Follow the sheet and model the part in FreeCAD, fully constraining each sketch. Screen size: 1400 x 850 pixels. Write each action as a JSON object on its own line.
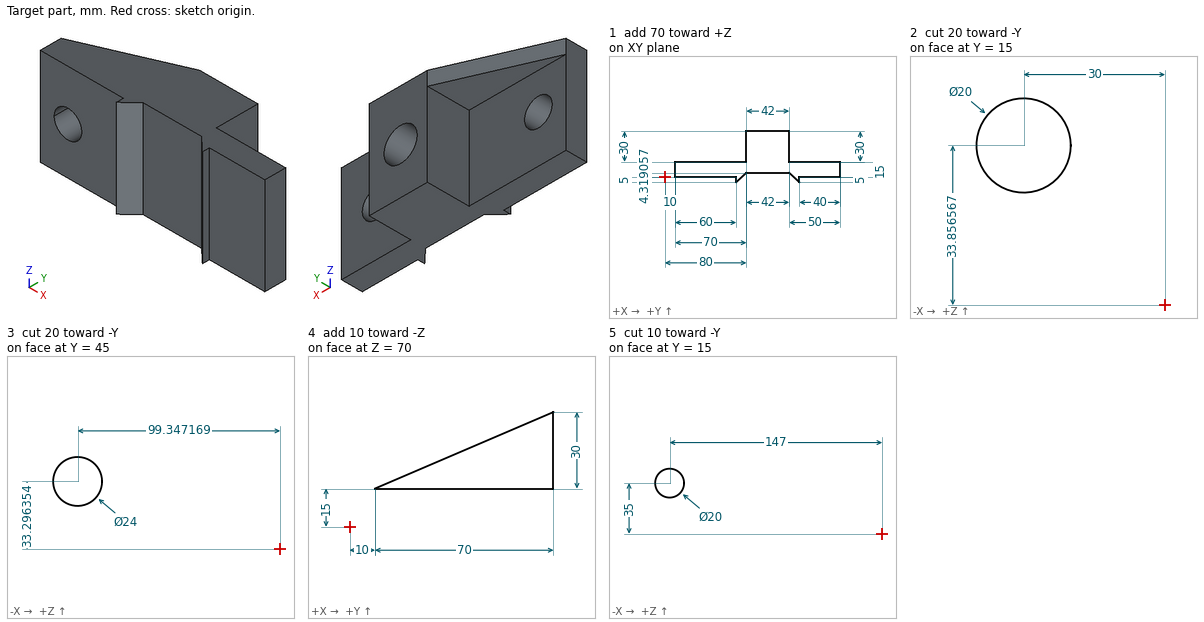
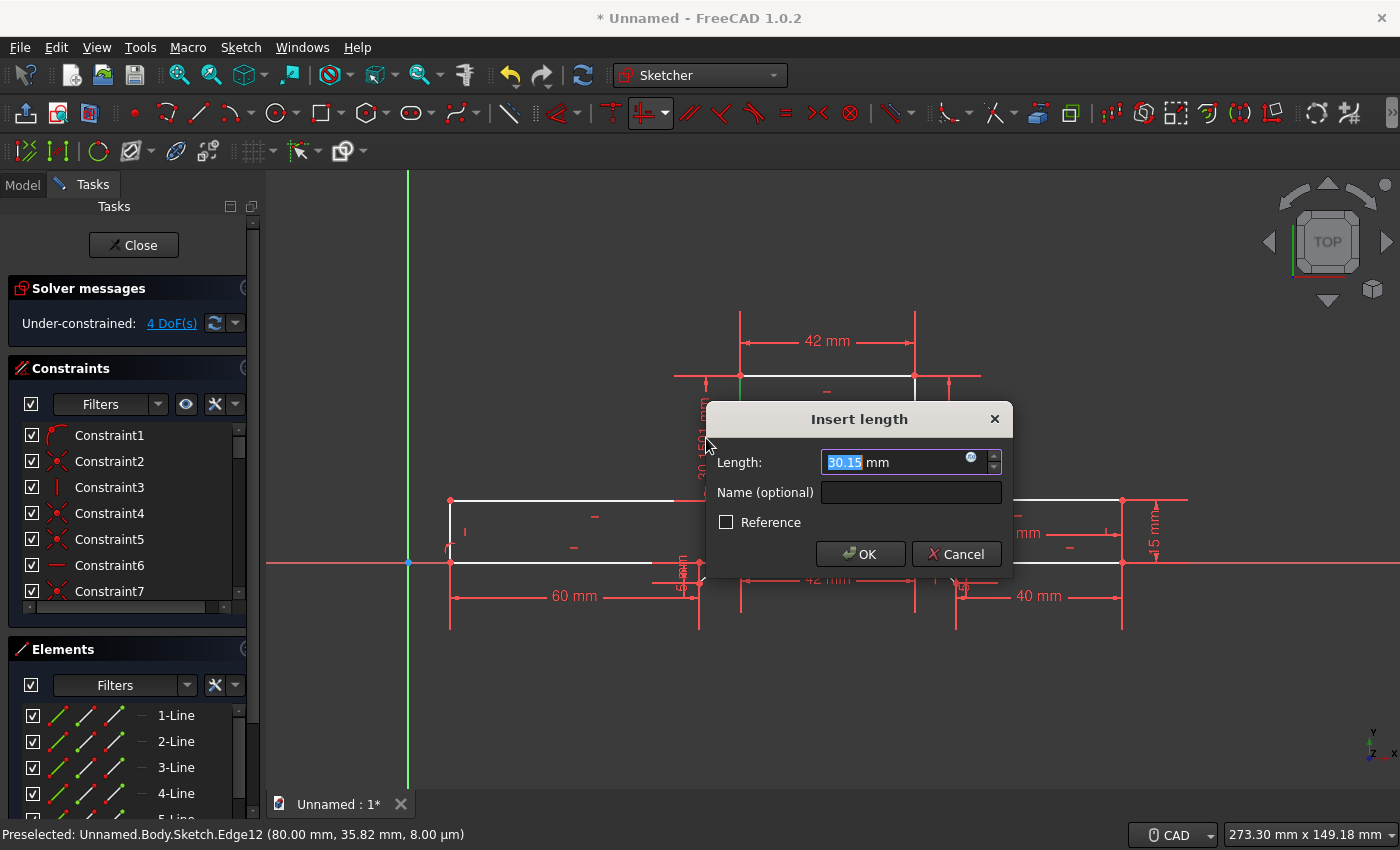
{"action": "type", "text": "30"}
{"action": "key", "text": "Return"}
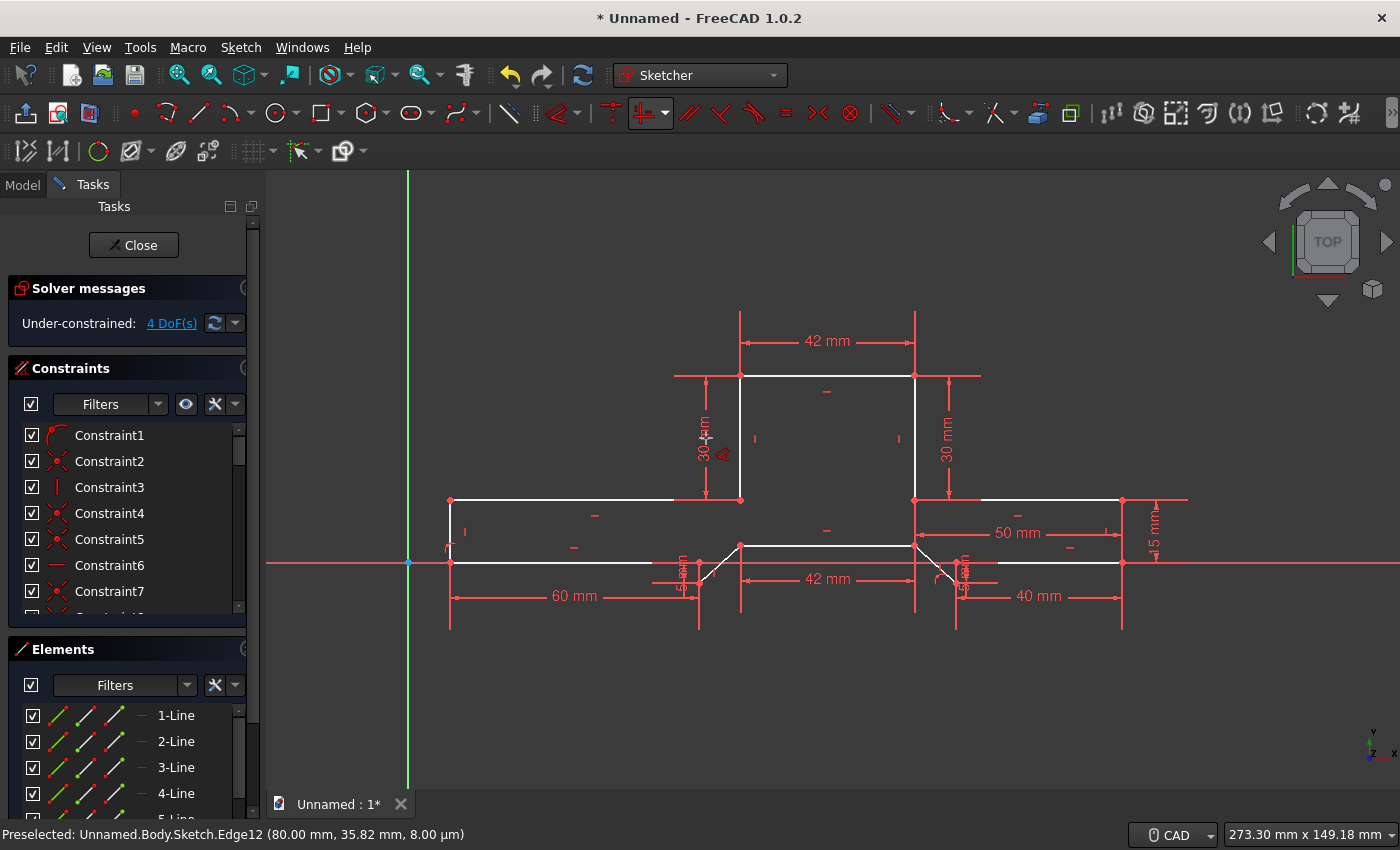
{"action": "left_click", "coordinate": [653, 500]}
{"action": "left_click", "coordinate": [595, 534]}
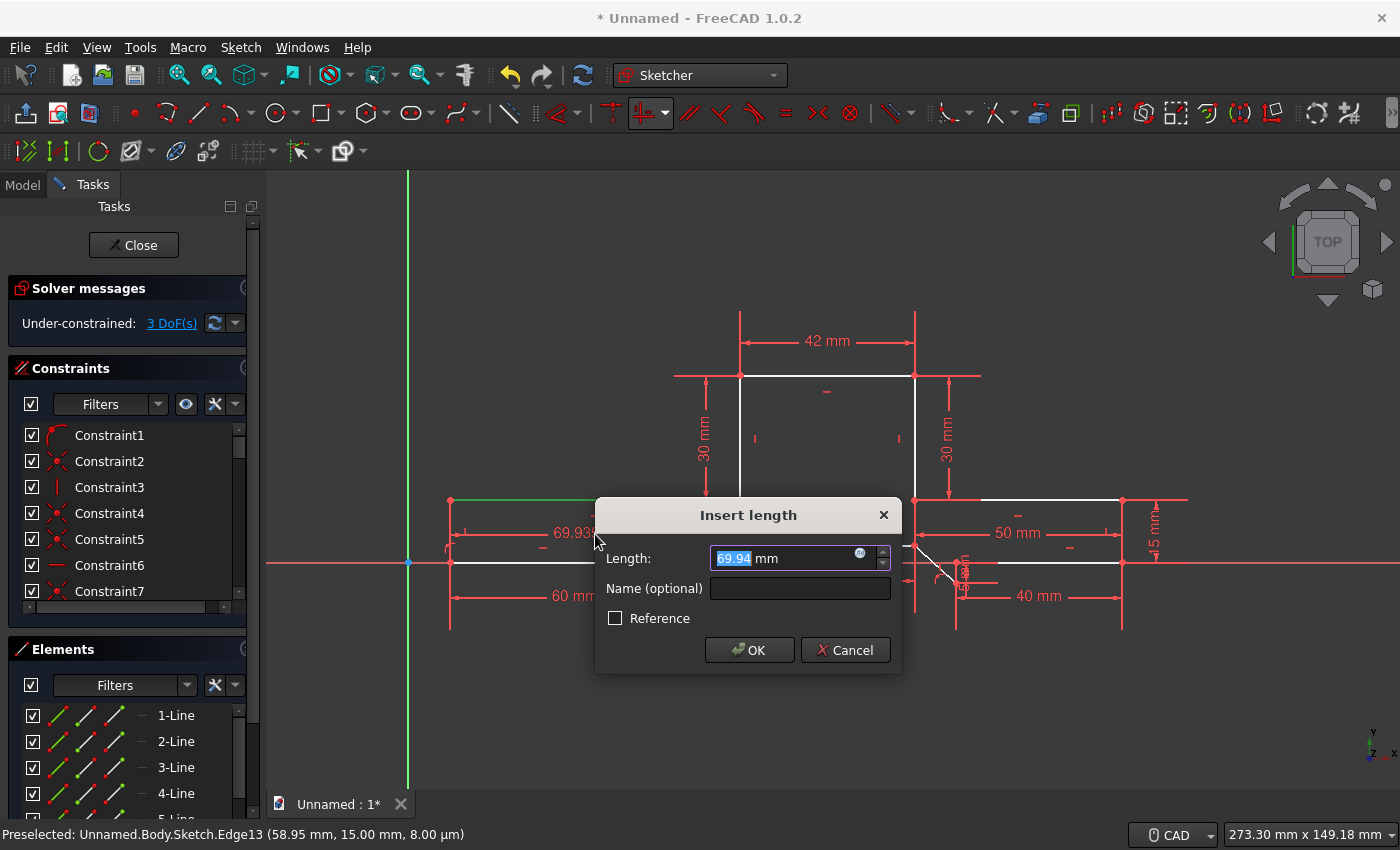
{"action": "type", "text": "70"}
{"action": "key", "text": "Return"}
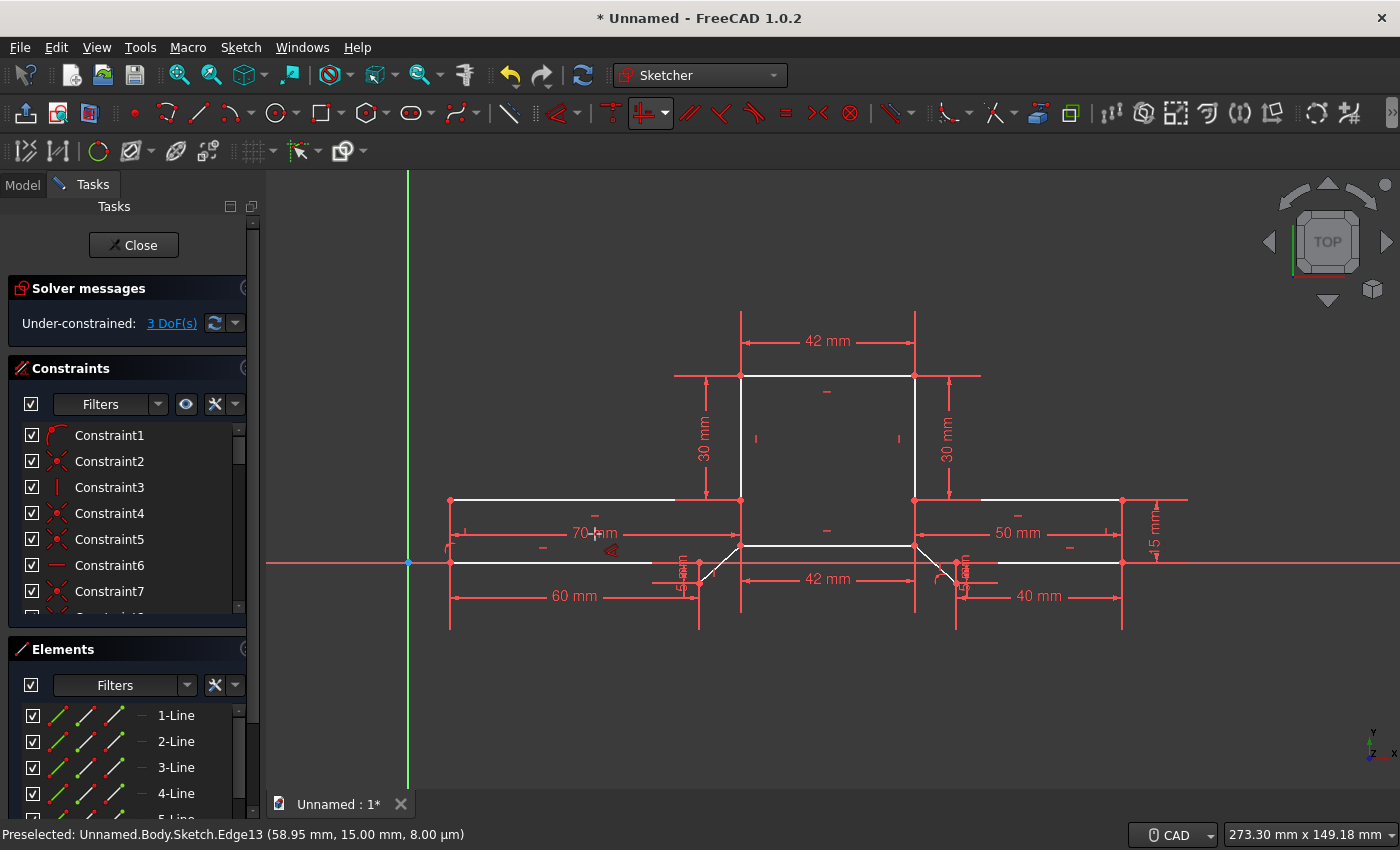
{"action": "left_click", "coordinate": [450, 563]}
{"action": "left_click", "coordinate": [429, 597]}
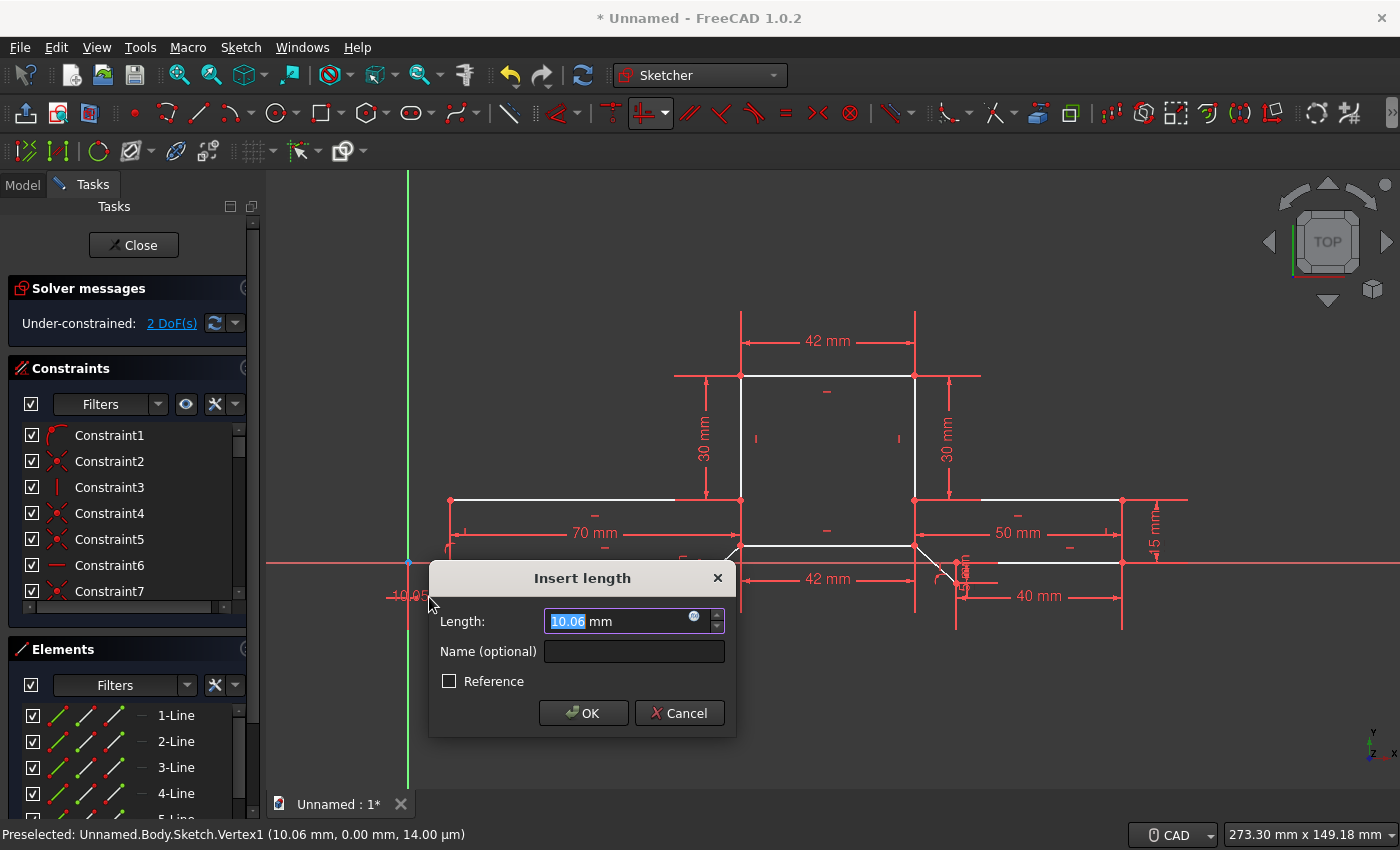
{"action": "type", "text": "10"}
{"action": "key", "text": "Return"}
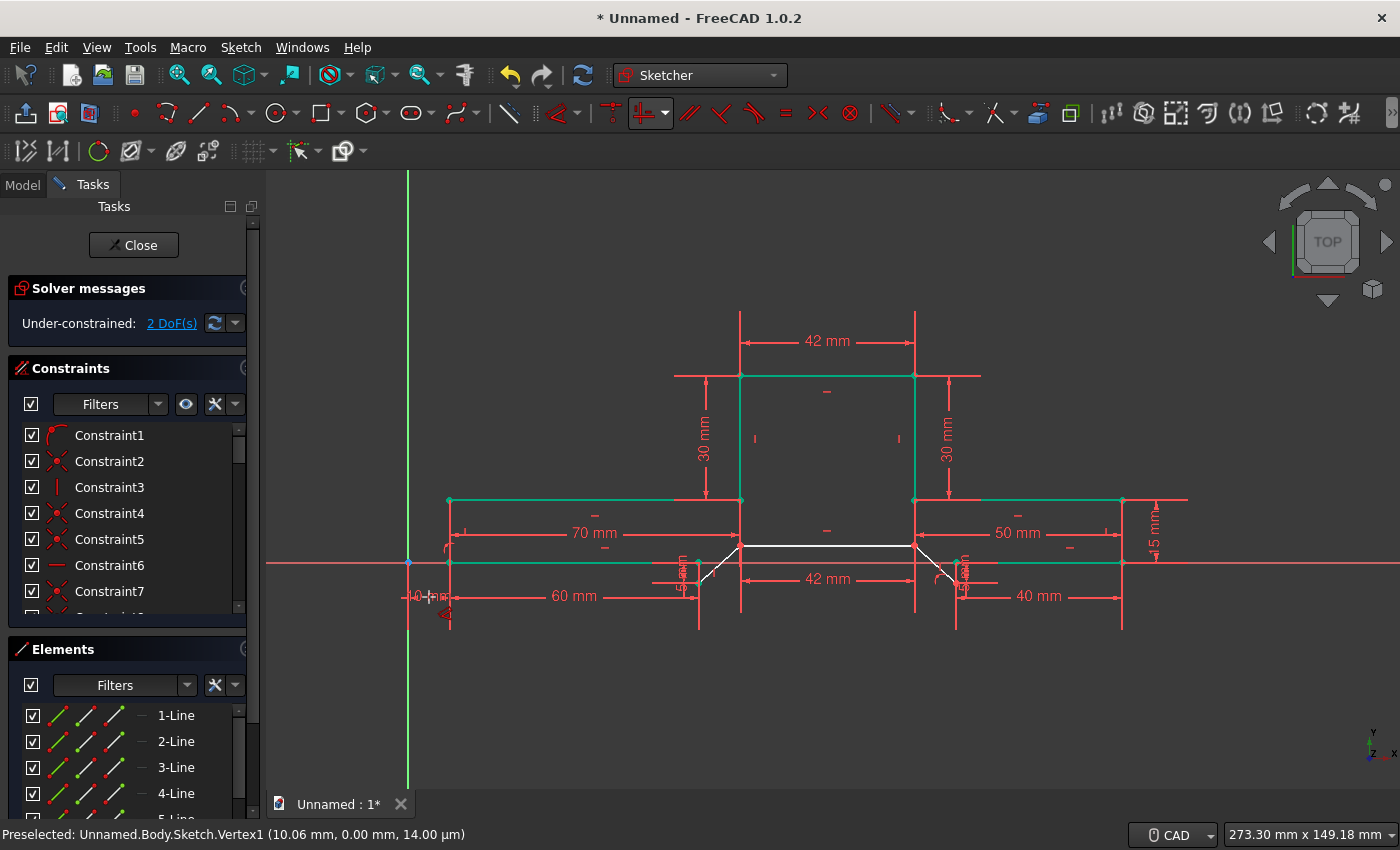
{"action": "left_click", "coordinate": [741, 546]}
{"action": "left_click", "coordinate": [651, 597]}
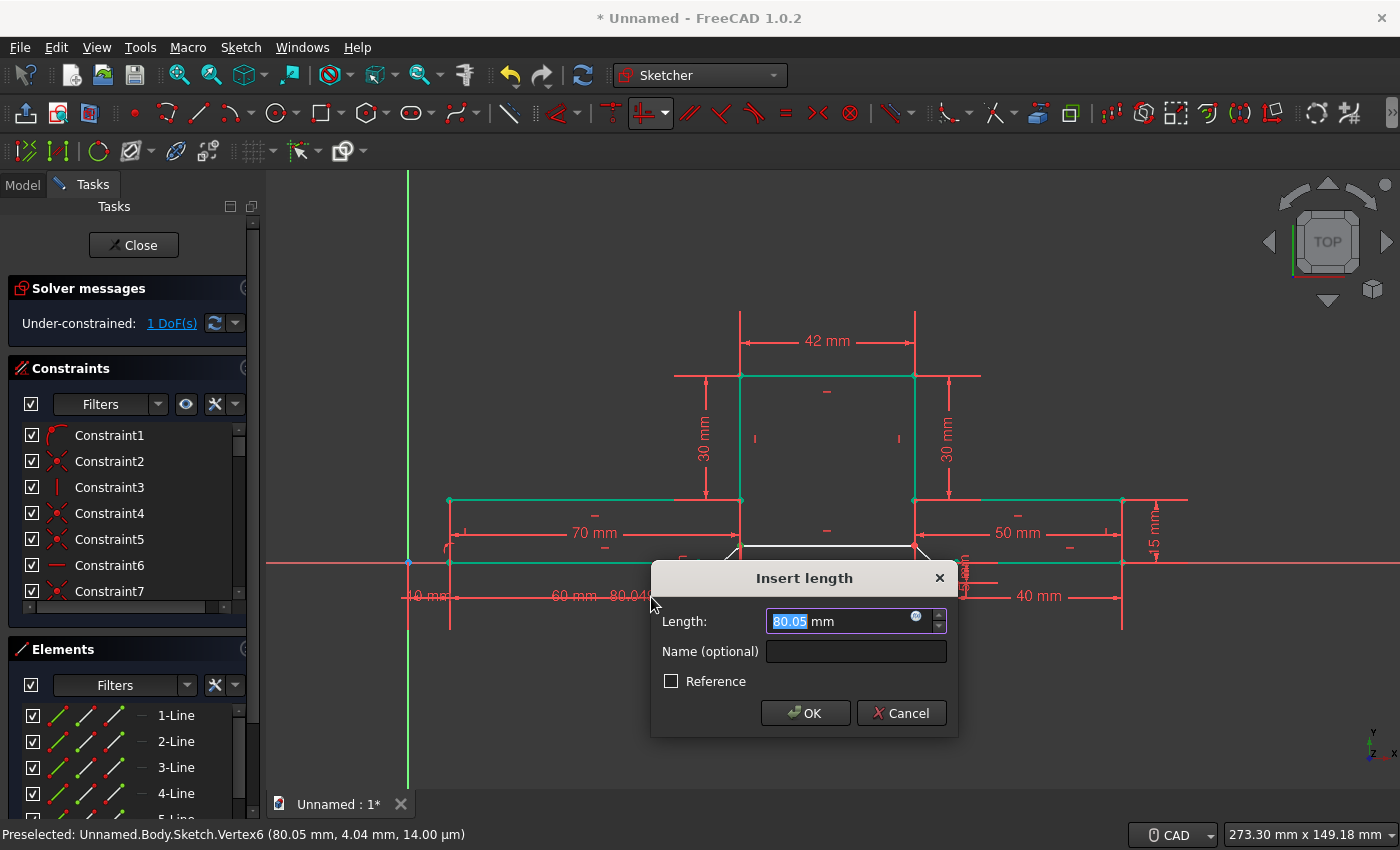
{"action": "type", "text": "80"}
{"action": "key", "text": "Return"}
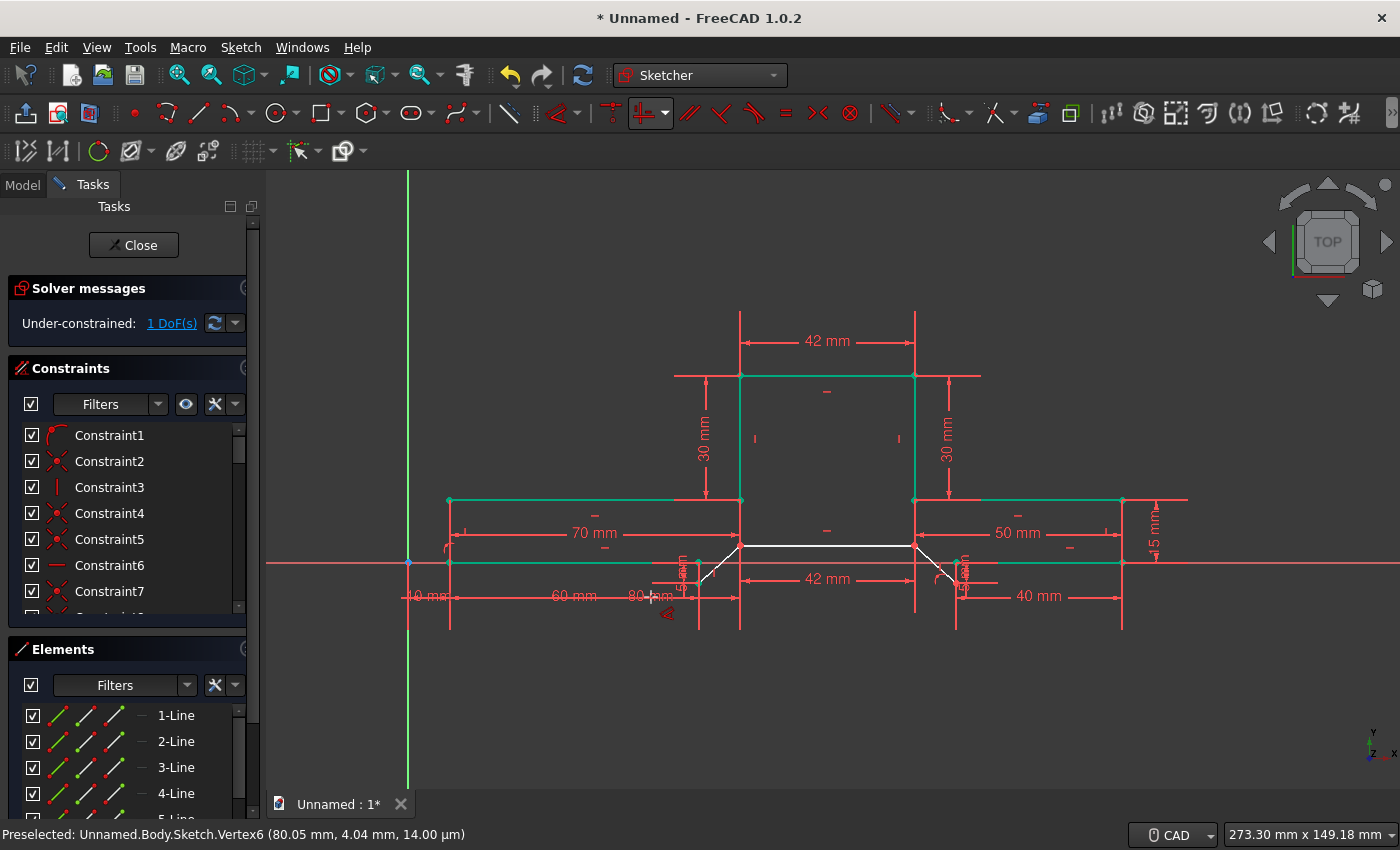
{"action": "scroll", "coordinate": [740, 546], "scroll_direction": "up", "scroll_amount": 4}